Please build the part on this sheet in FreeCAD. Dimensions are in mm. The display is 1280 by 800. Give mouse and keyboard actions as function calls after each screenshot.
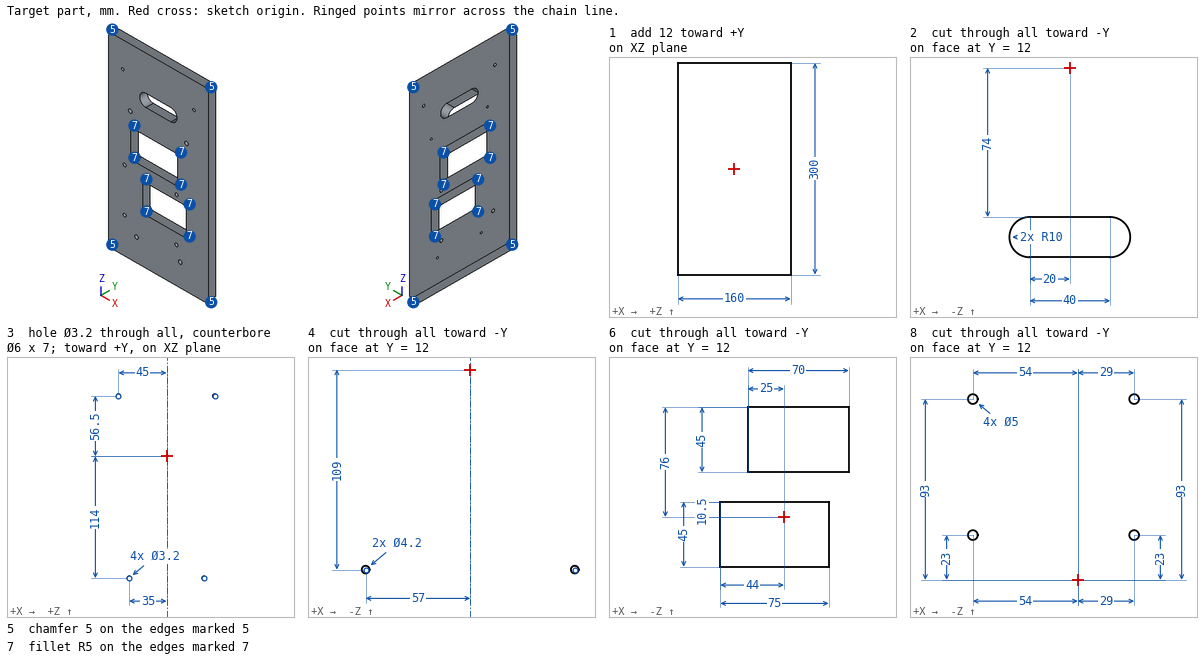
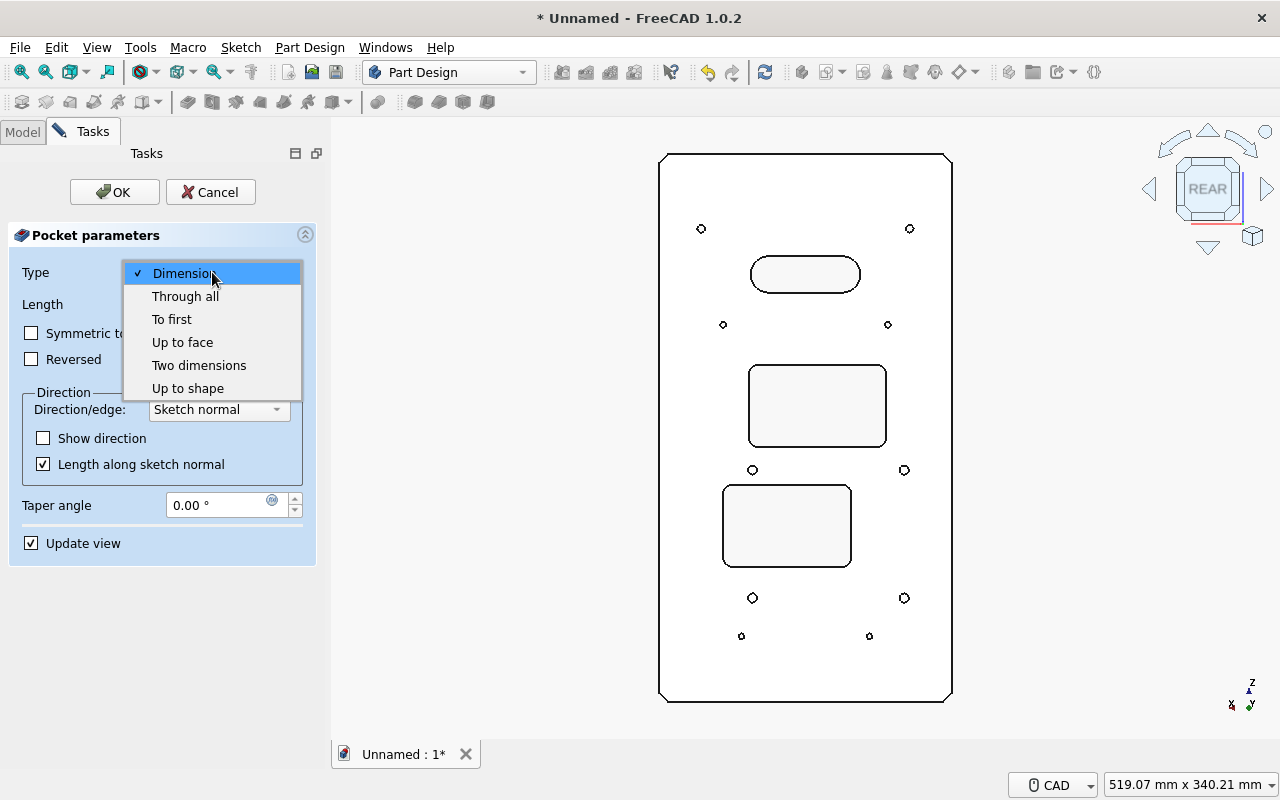
click(212, 296)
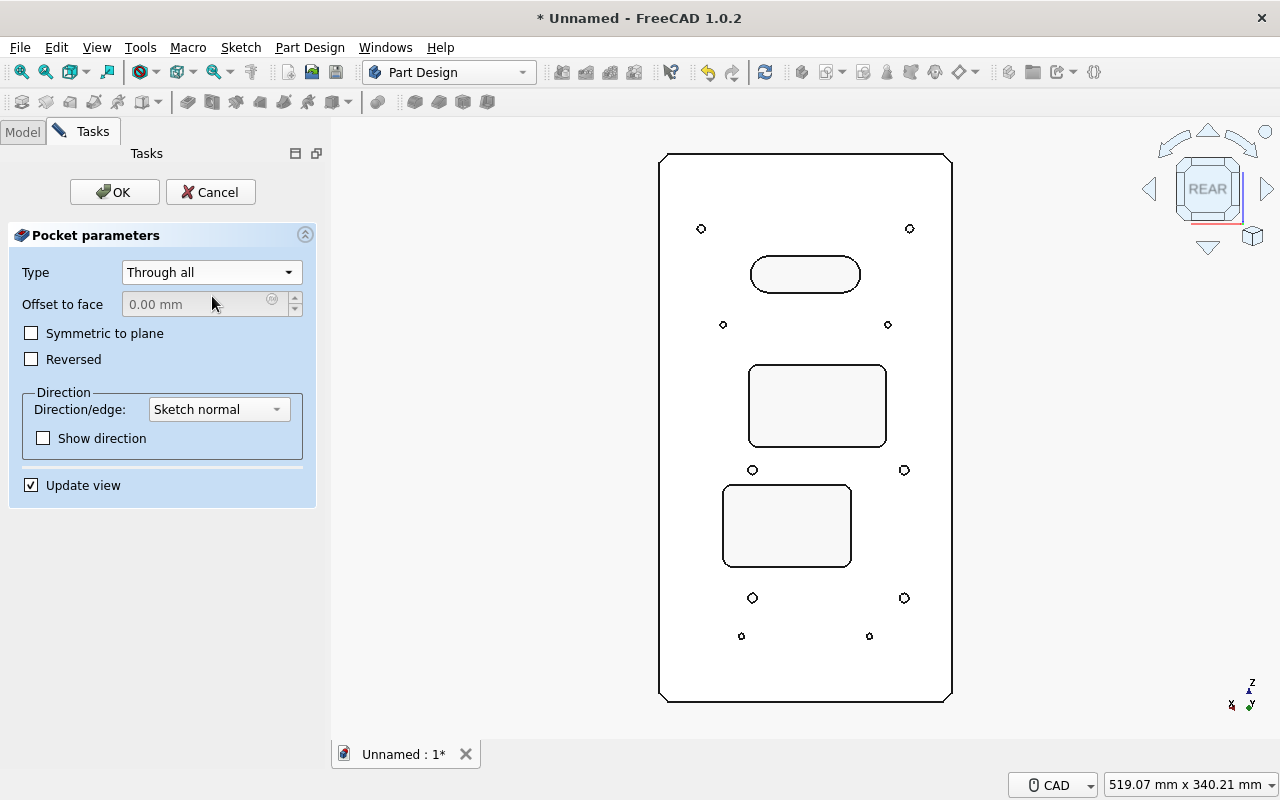
click(115, 192)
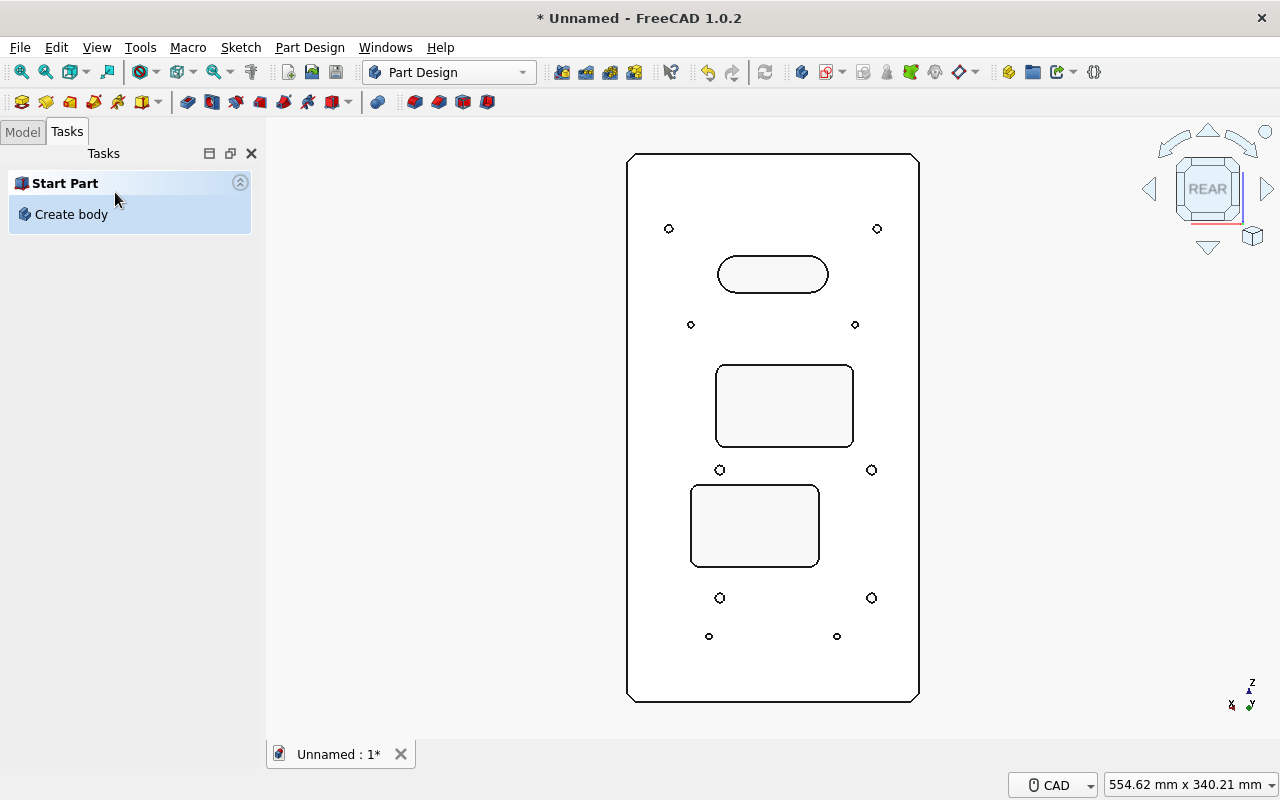
key(0)